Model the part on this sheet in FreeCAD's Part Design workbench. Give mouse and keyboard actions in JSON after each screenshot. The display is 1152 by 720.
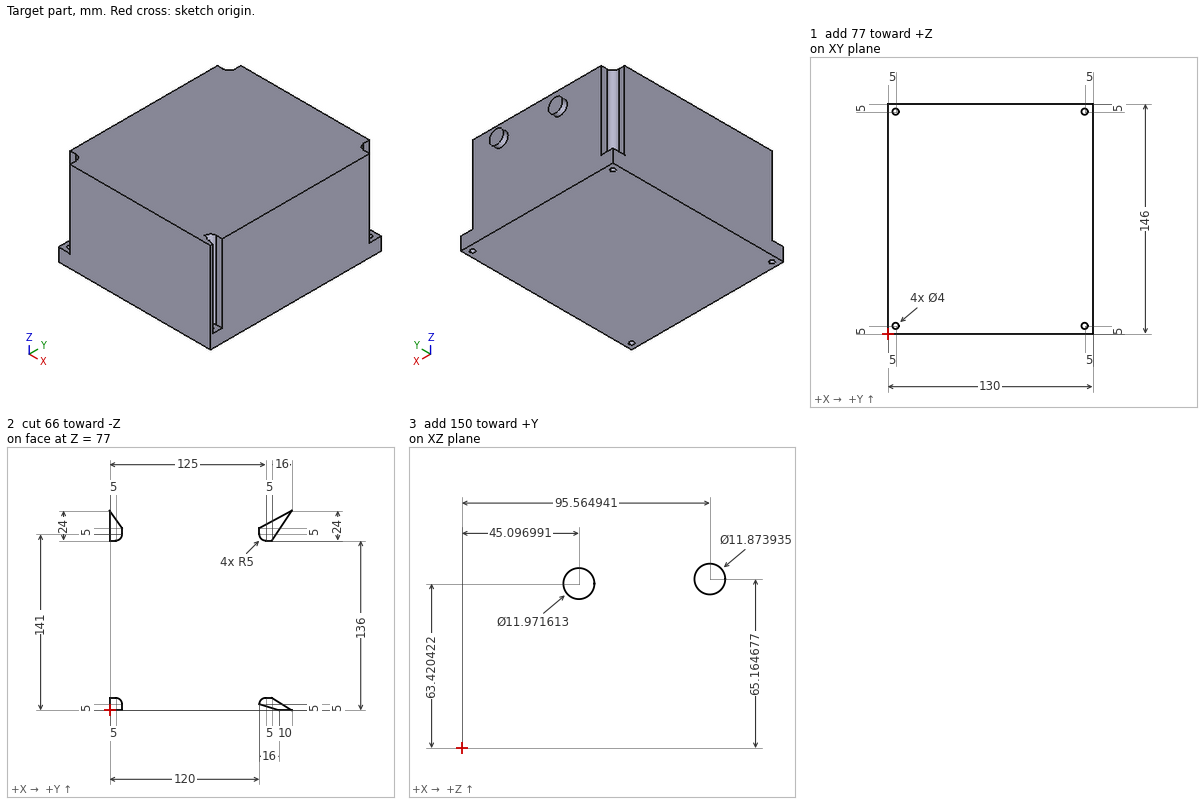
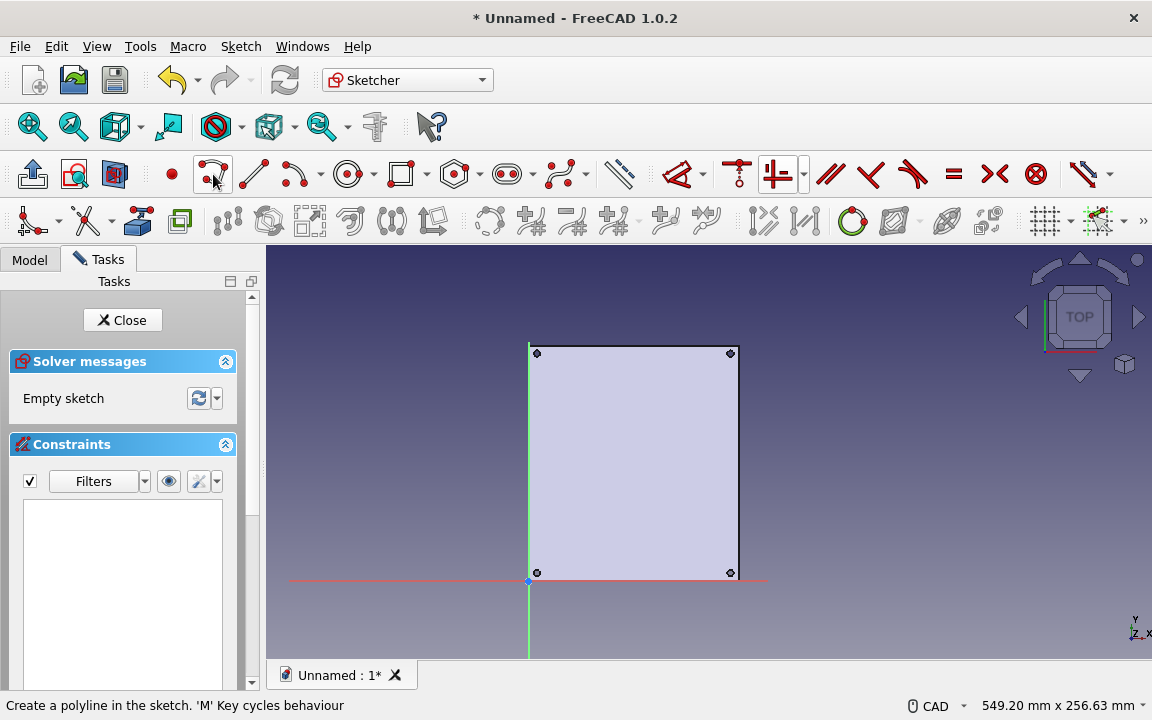
{"action": "left_click", "coordinate": [731, 362]}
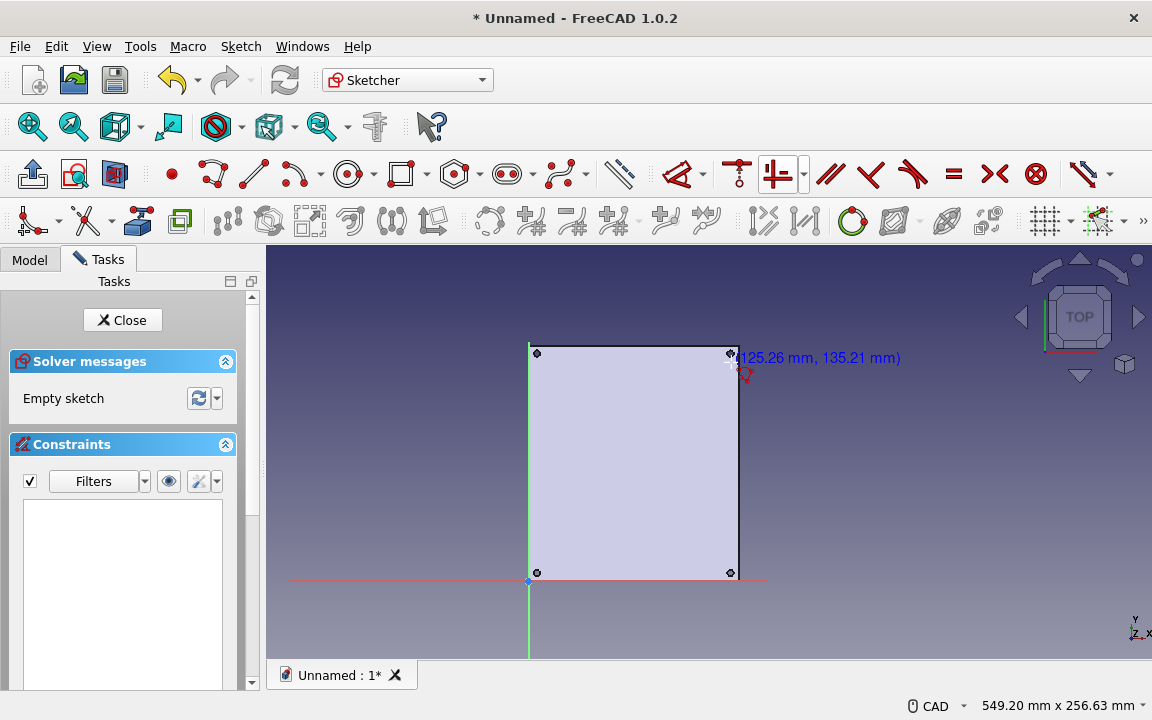
{"action": "scroll", "coordinate": [739, 362], "scroll_direction": "up", "scroll_amount": 4}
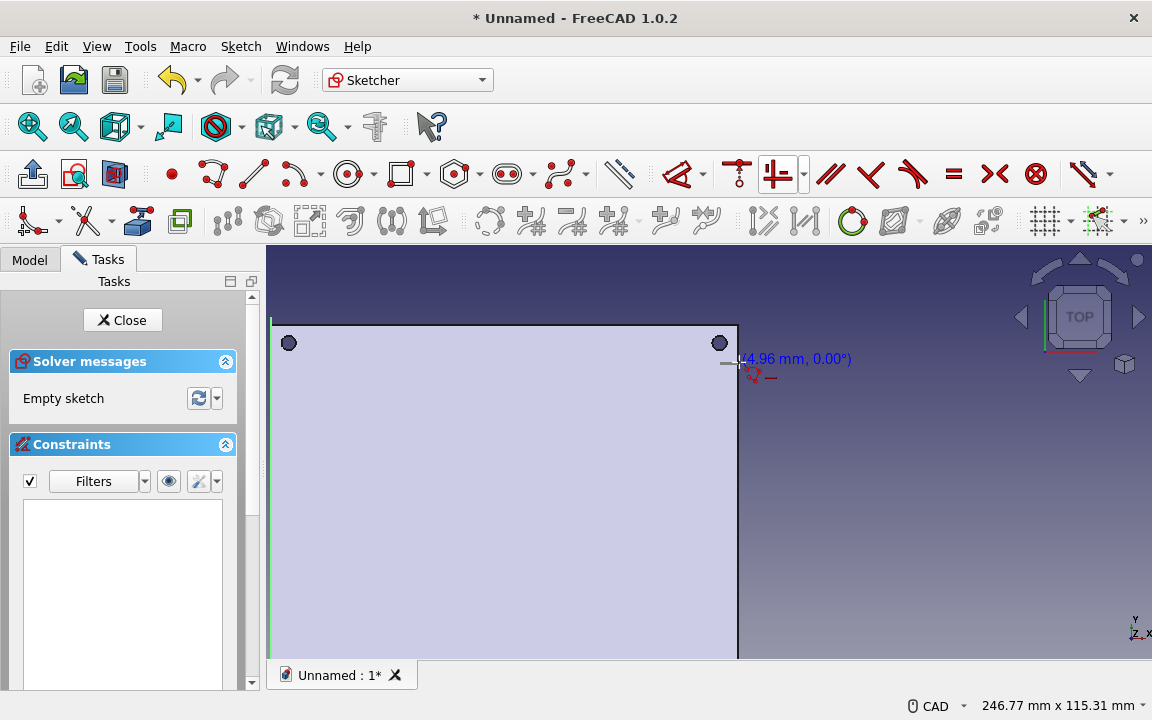
{"action": "left_click", "coordinate": [738, 362]}
{"action": "left_click", "coordinate": [795, 275]}
{"action": "left_click", "coordinate": [702, 325]}
{"action": "left_click", "coordinate": [702, 343]}
{"action": "right_click", "coordinate": [702, 343]}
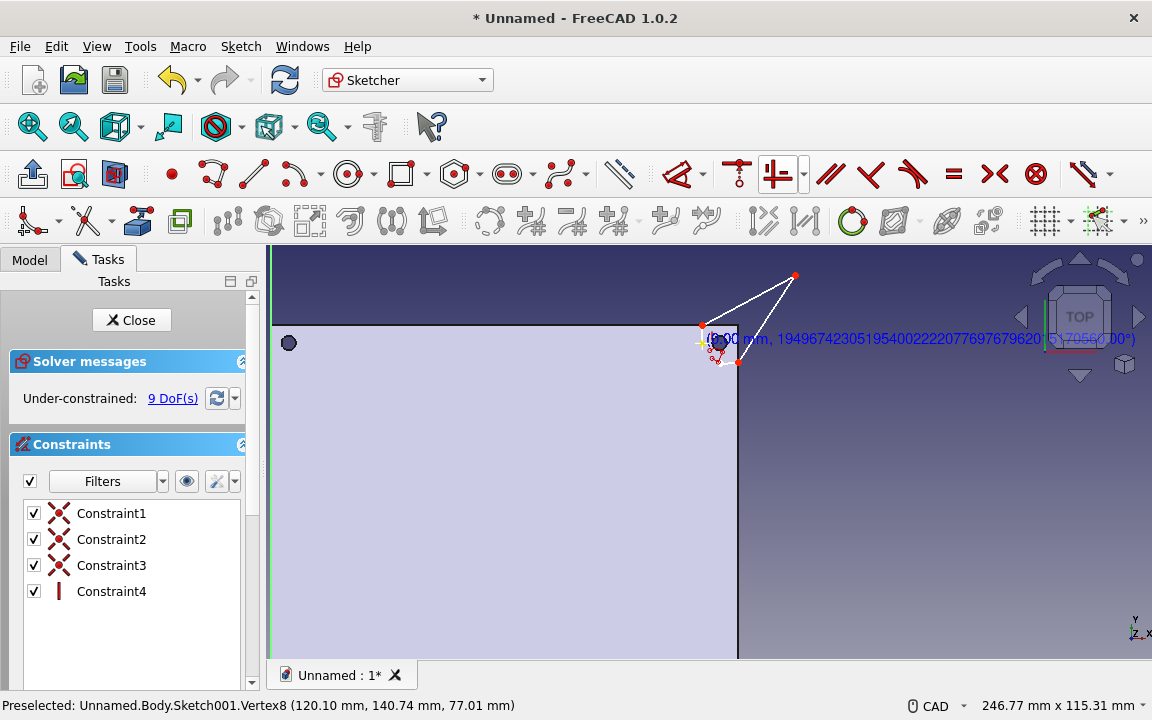
{"action": "left_click", "coordinate": [320, 174]}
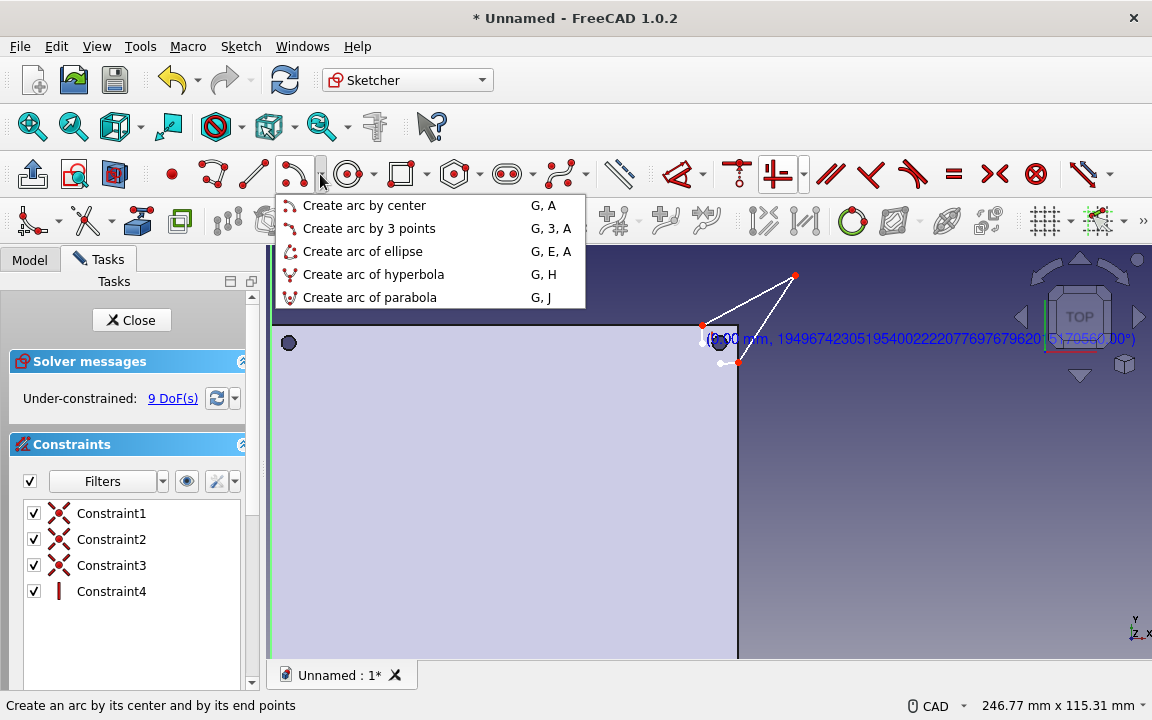
{"action": "left_click", "coordinate": [430, 228]}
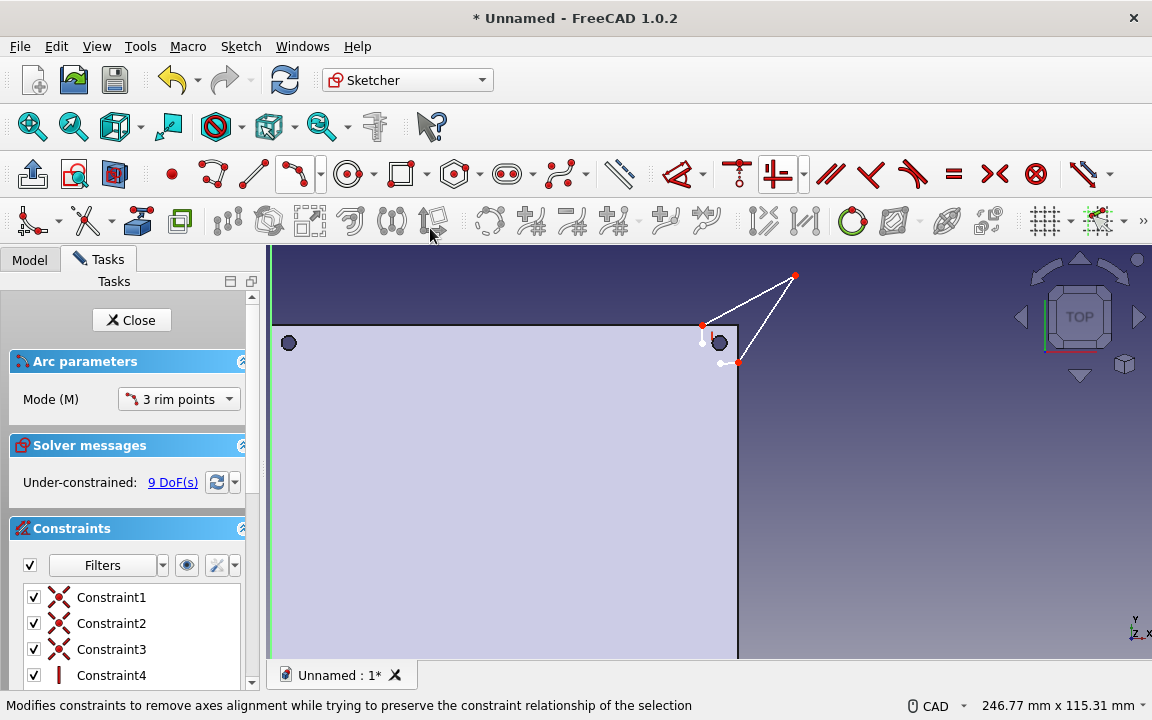
{"action": "scroll", "coordinate": [702, 343], "scroll_direction": "up", "scroll_amount": 3}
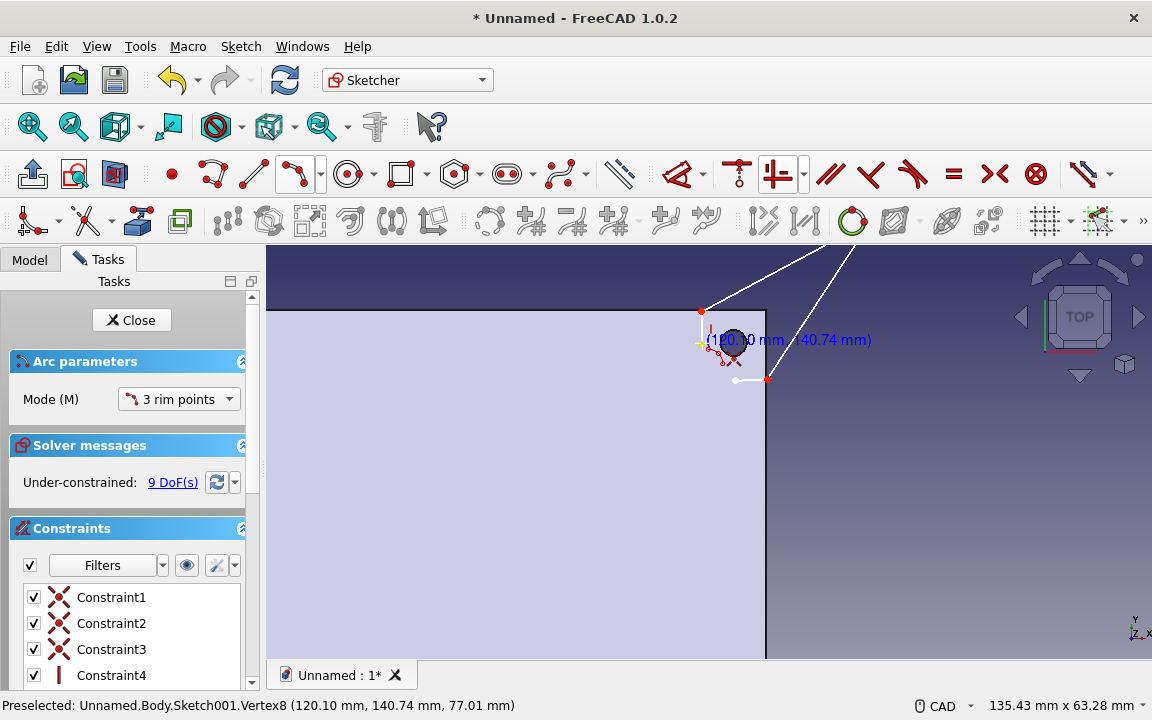
{"action": "left_click", "coordinate": [702, 345]}
{"action": "left_click", "coordinate": [735, 381]}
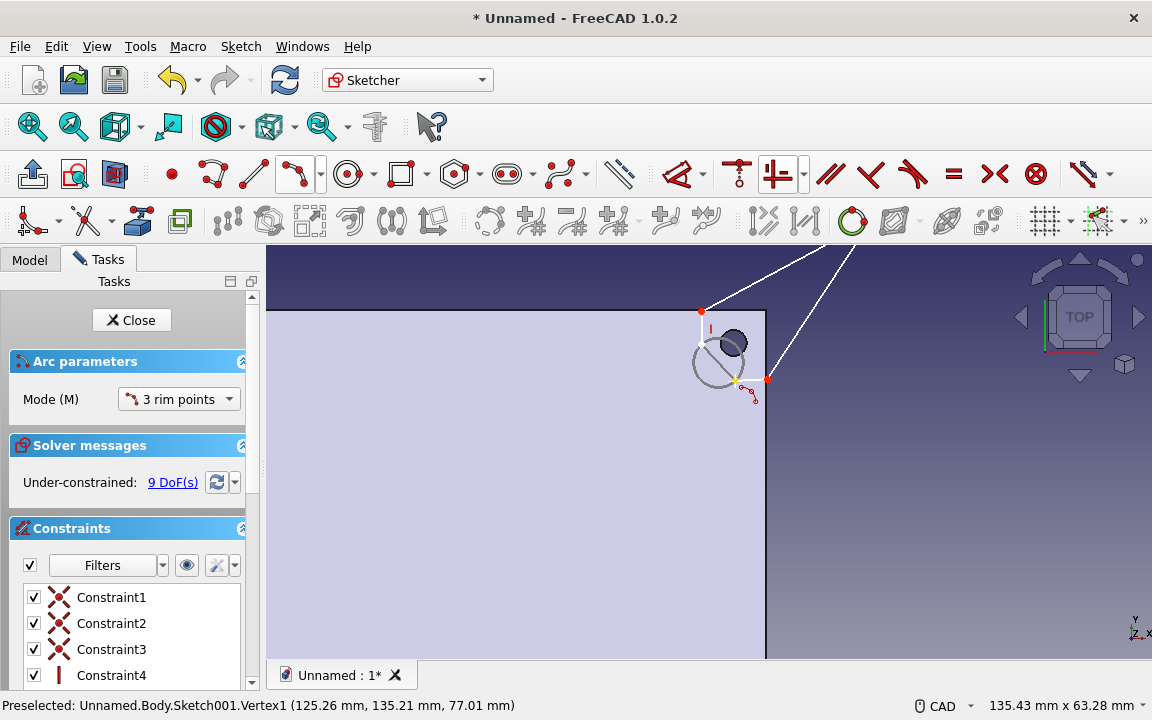
{"action": "scroll", "coordinate": [711, 366], "scroll_direction": "up", "scroll_amount": 3}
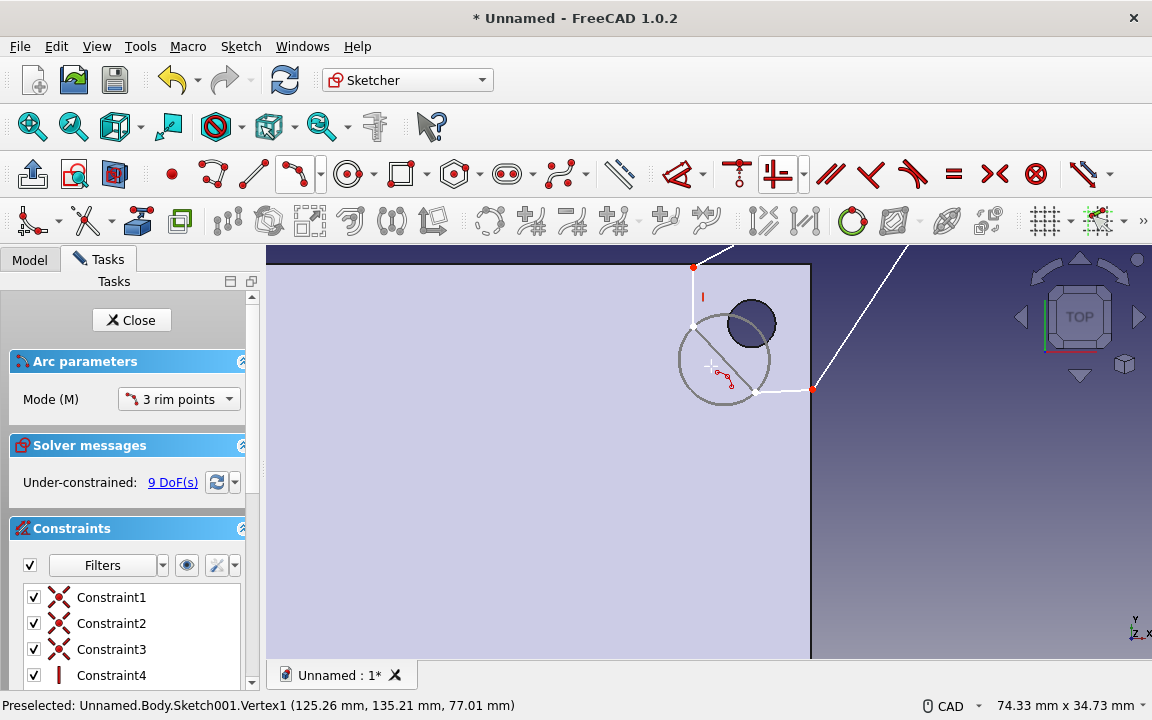
{"action": "left_click", "coordinate": [710, 366]}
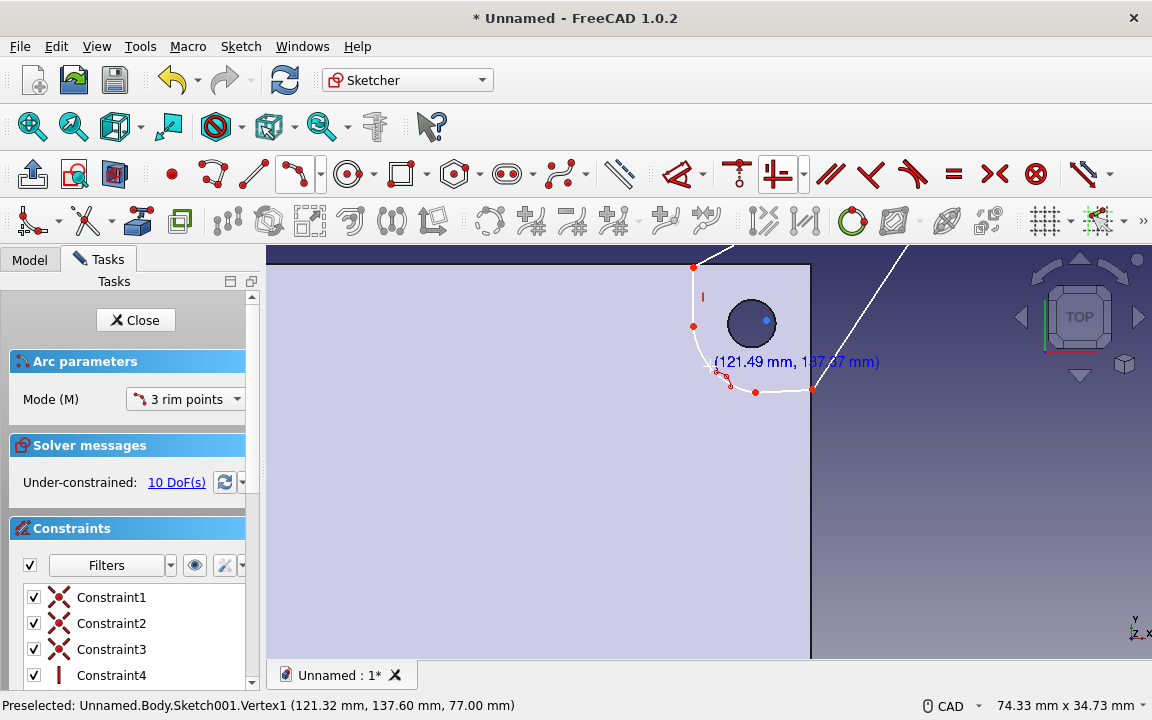
{"action": "left_click", "coordinate": [213, 174]}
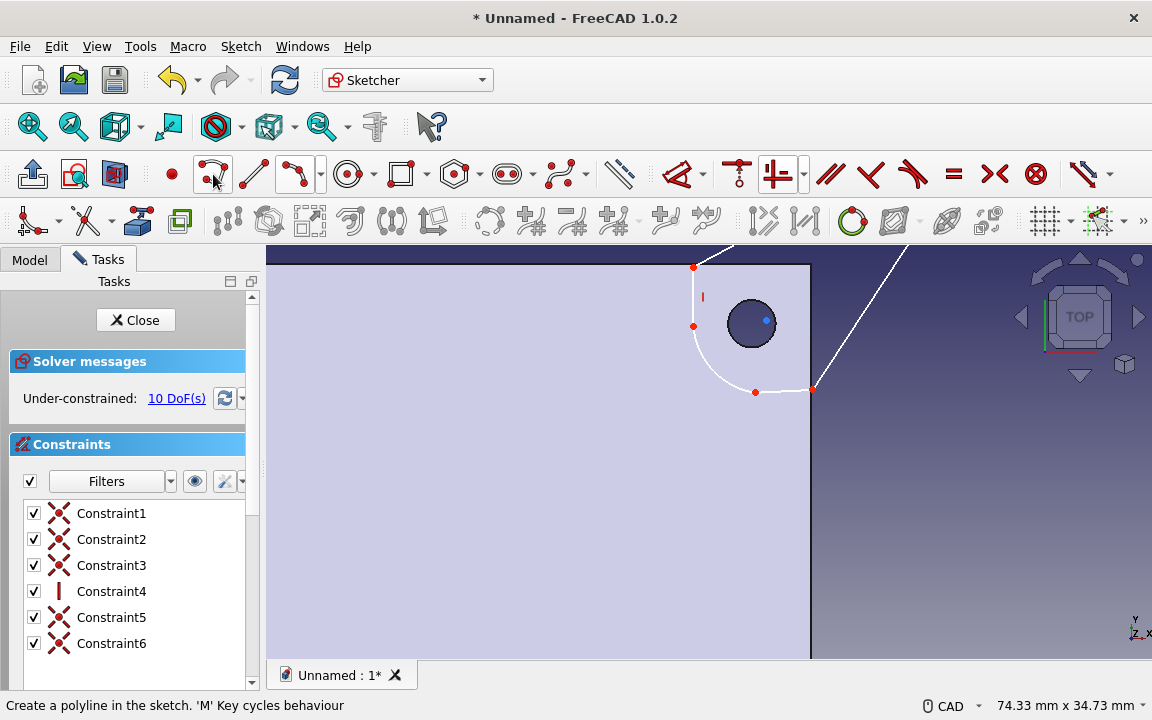
{"action": "scroll", "coordinate": [720, 358], "scroll_direction": "down", "scroll_amount": 10}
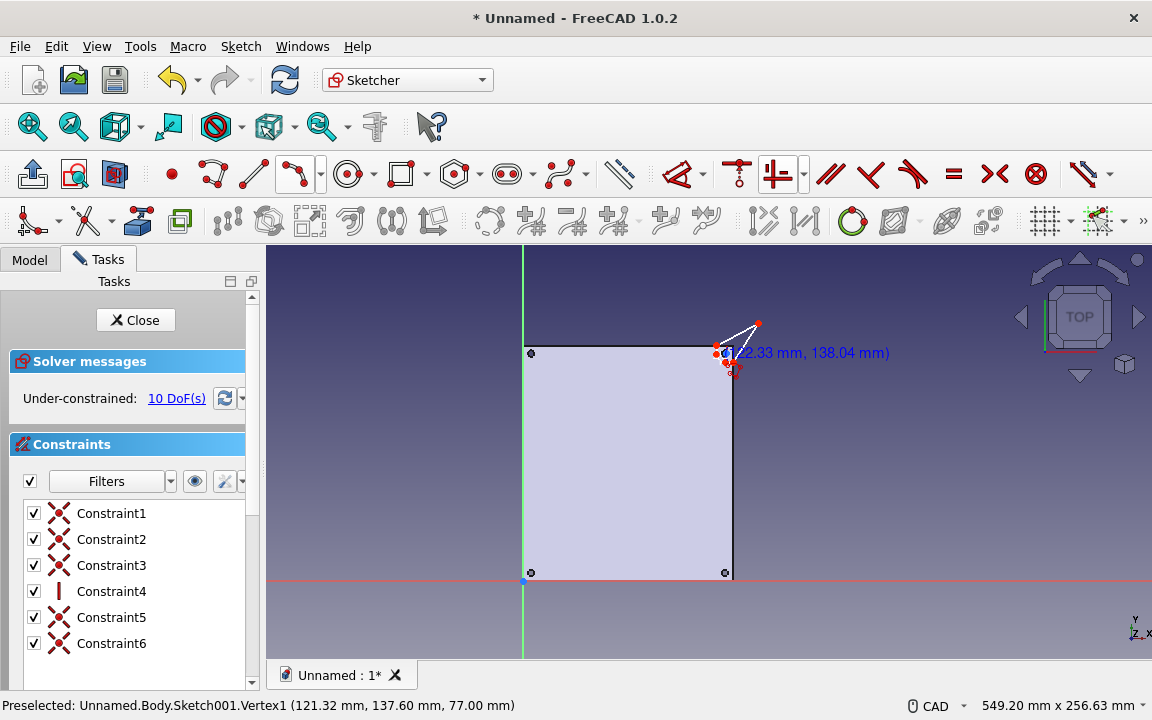
{"action": "left_click", "coordinate": [539, 354]}